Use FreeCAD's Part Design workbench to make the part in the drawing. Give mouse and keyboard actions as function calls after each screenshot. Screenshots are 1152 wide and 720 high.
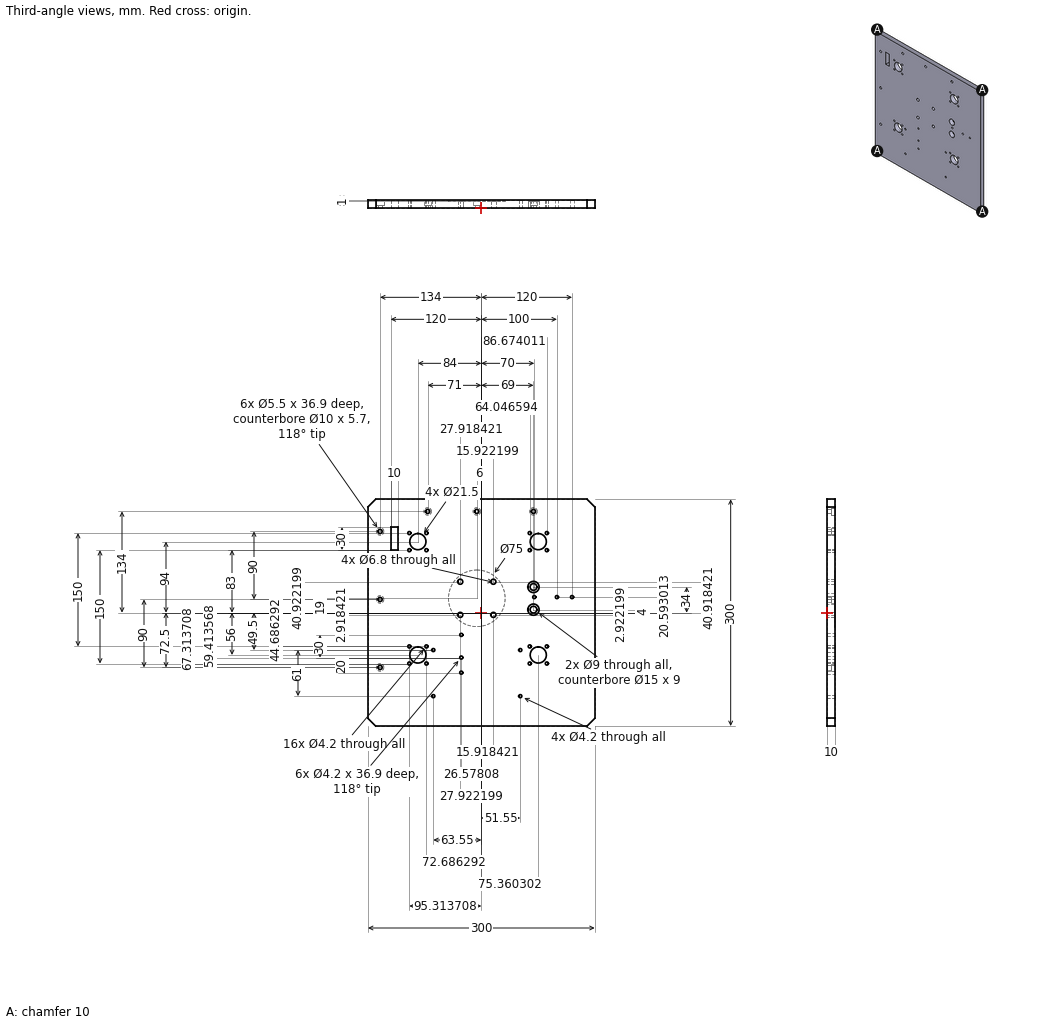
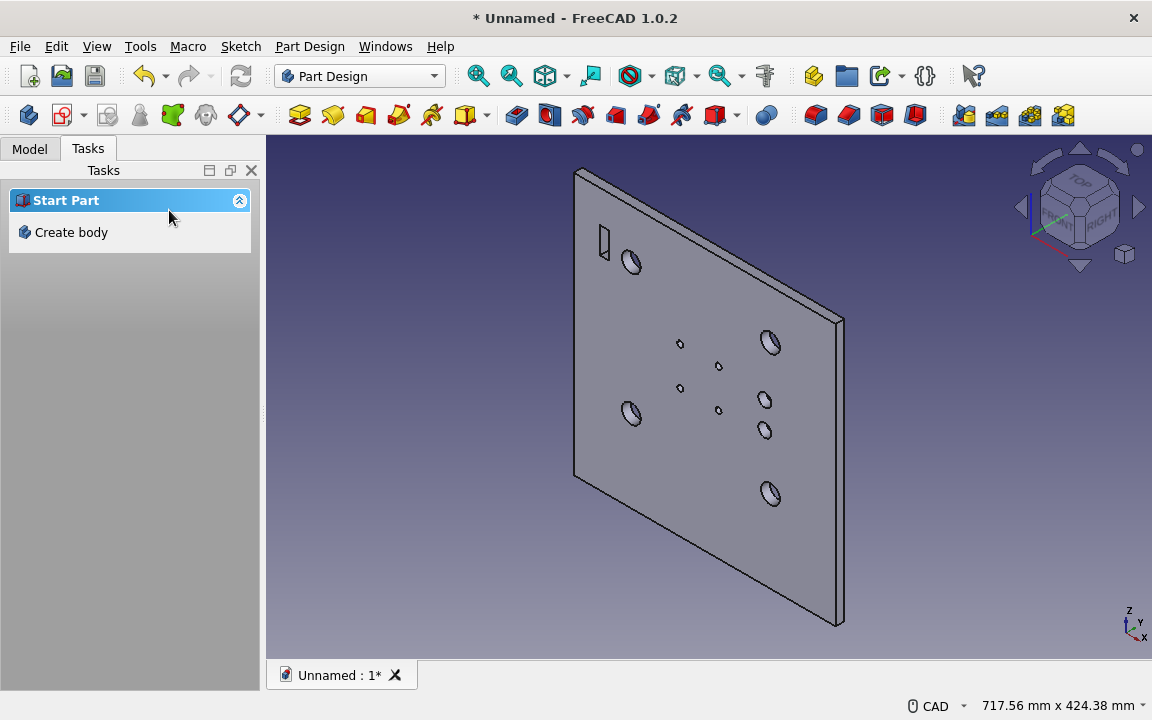
click(705, 485)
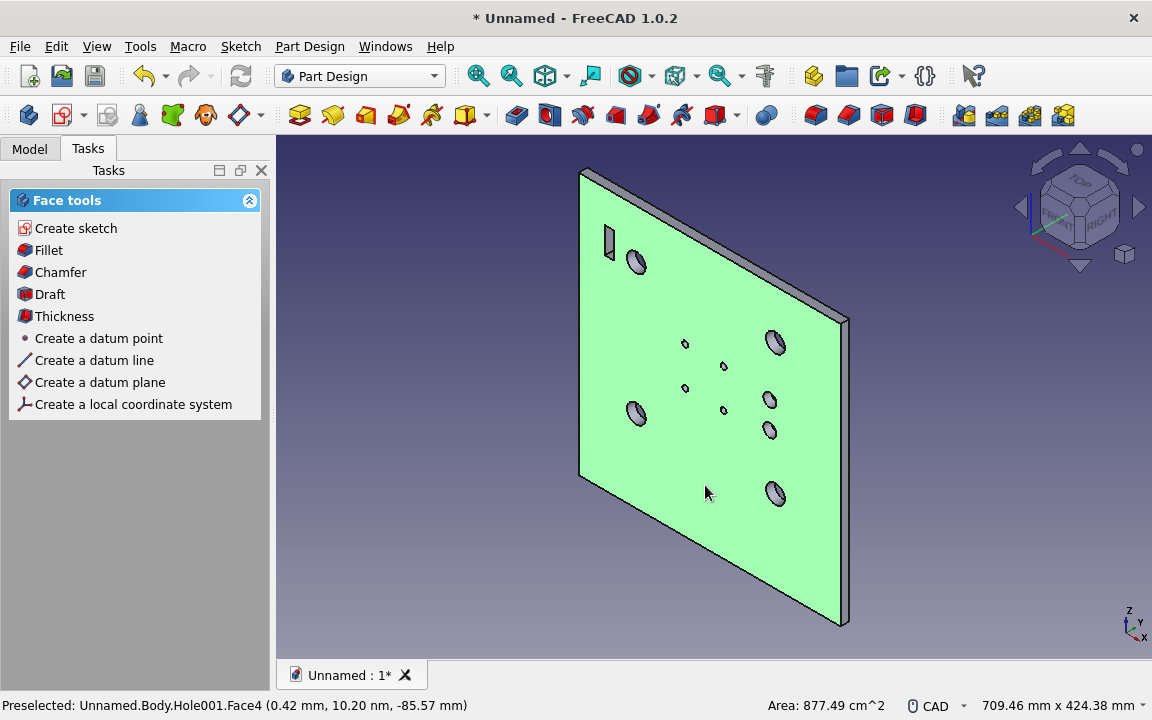
click(62, 116)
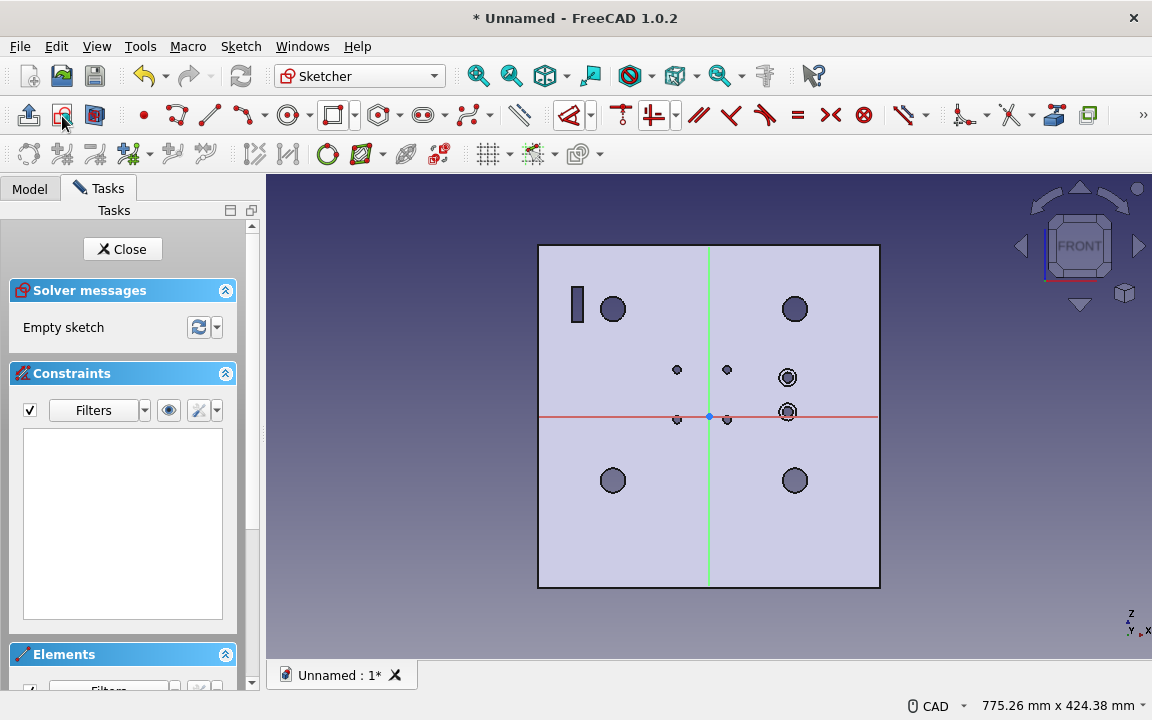
scroll(833, 351, up, 2)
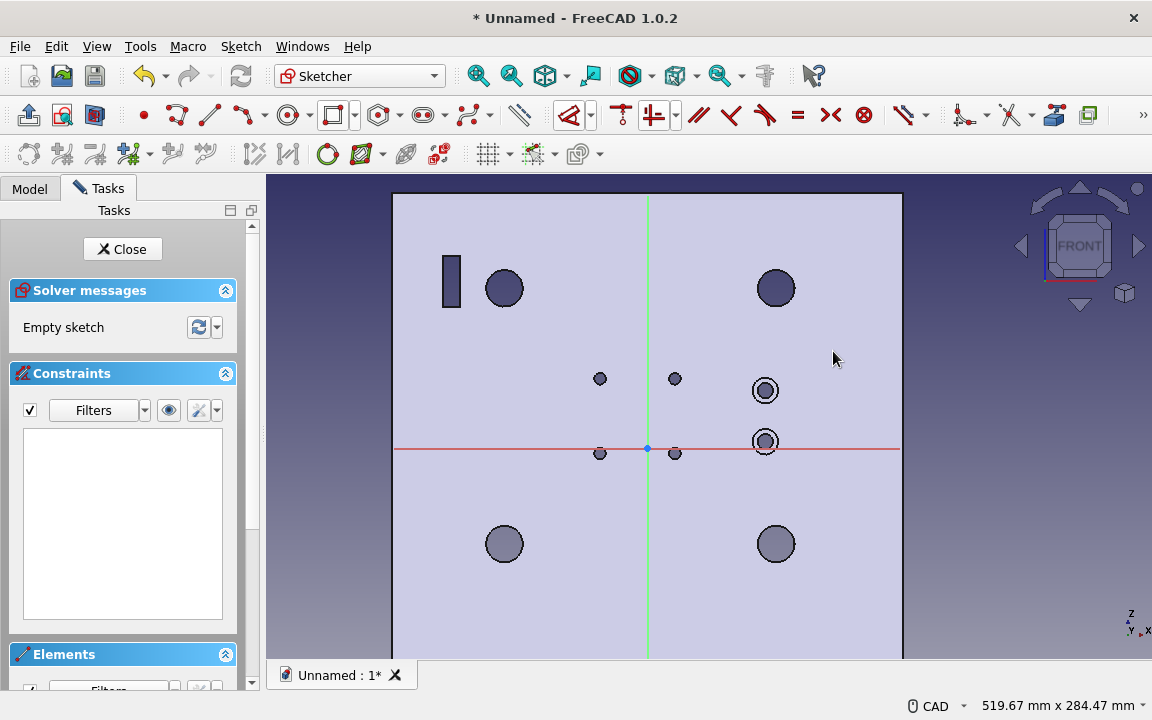
click(288, 116)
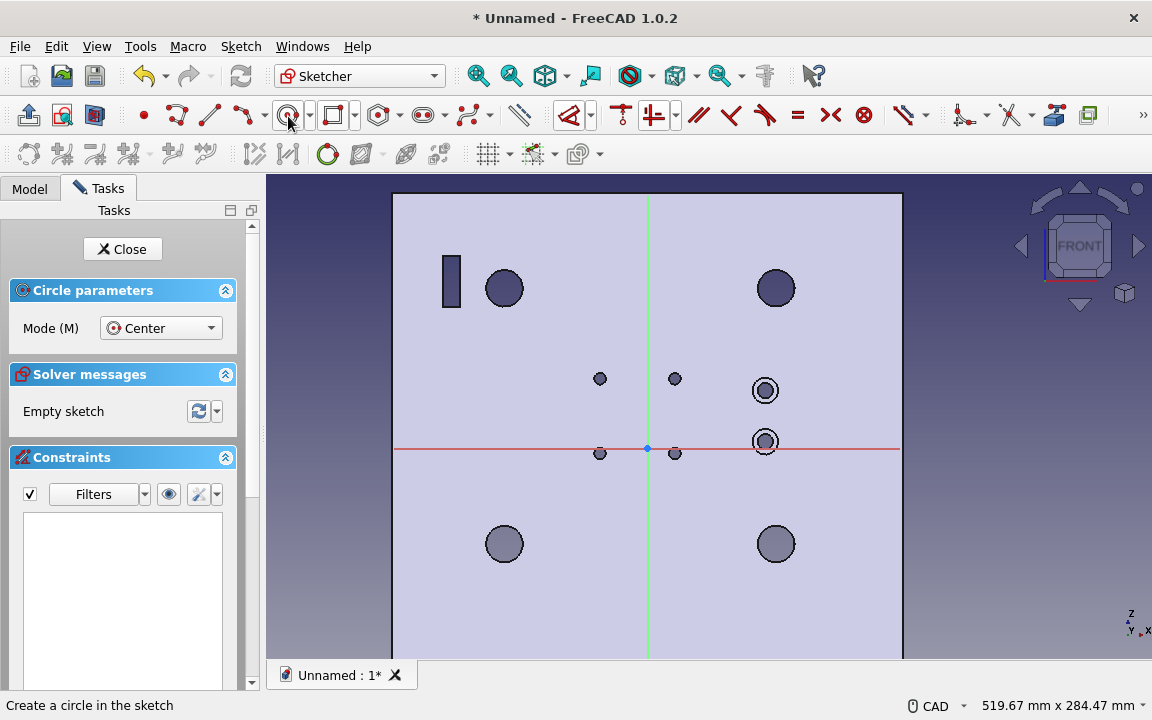
scroll(524, 525, up, 10)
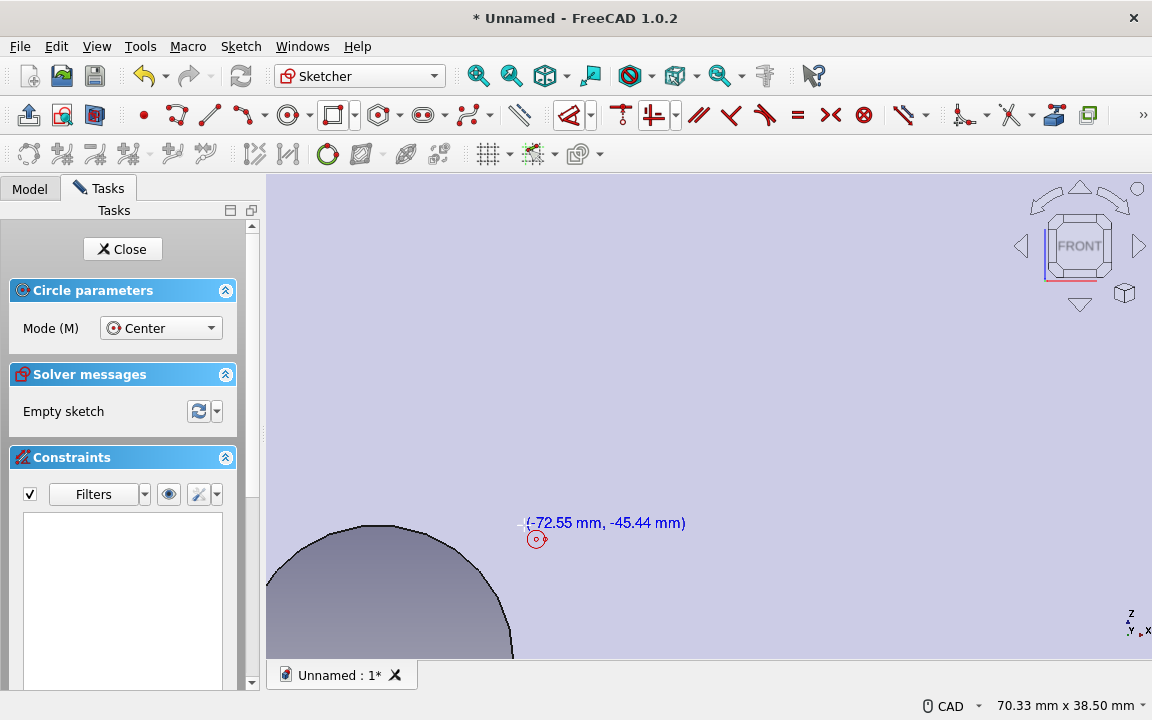
scroll(524, 526, down, 10)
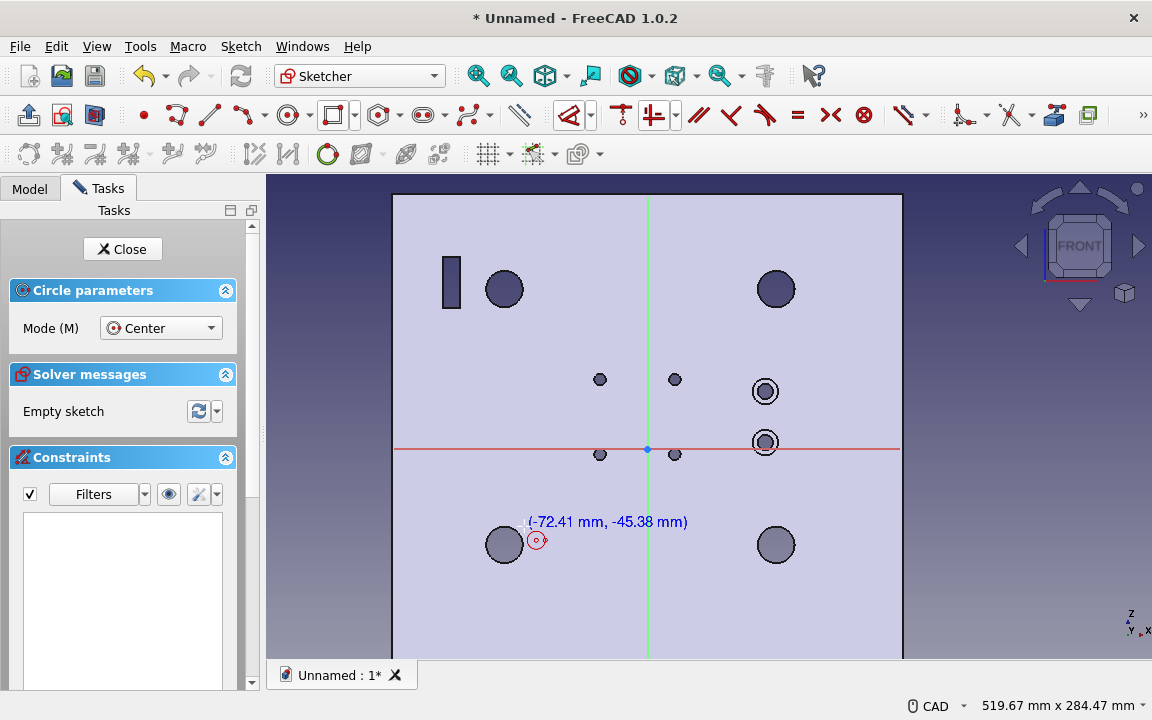
click(524, 526)
move(526, 523)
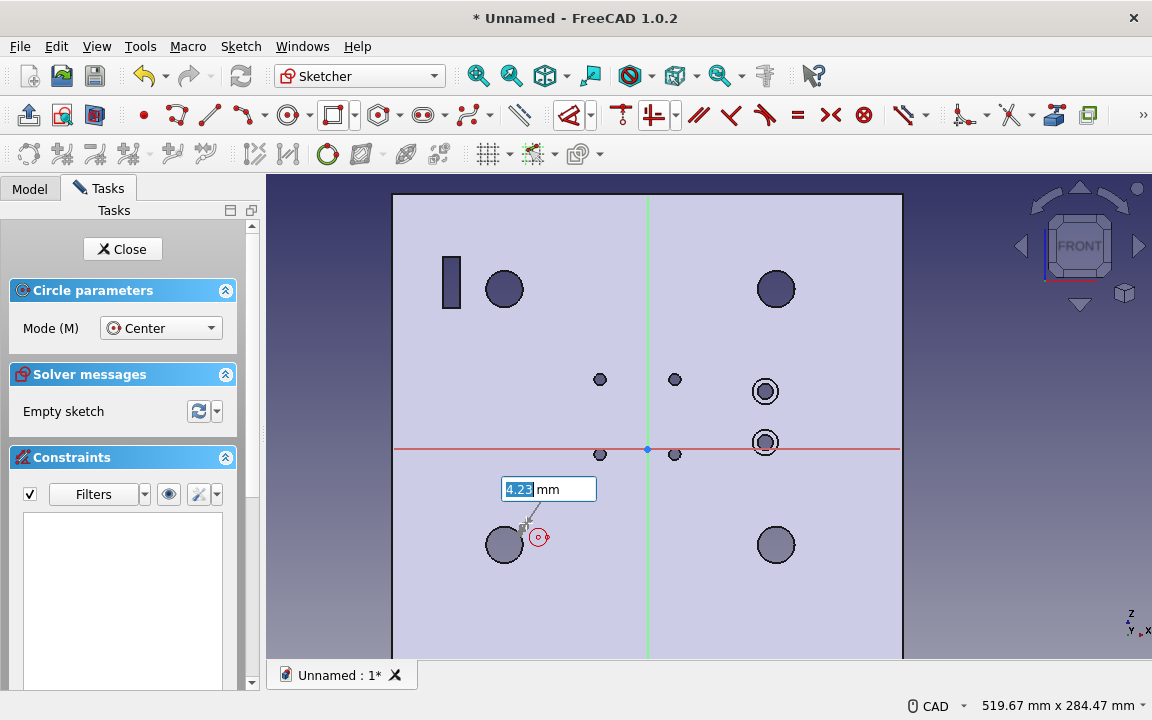
text(4.2)
key(Return)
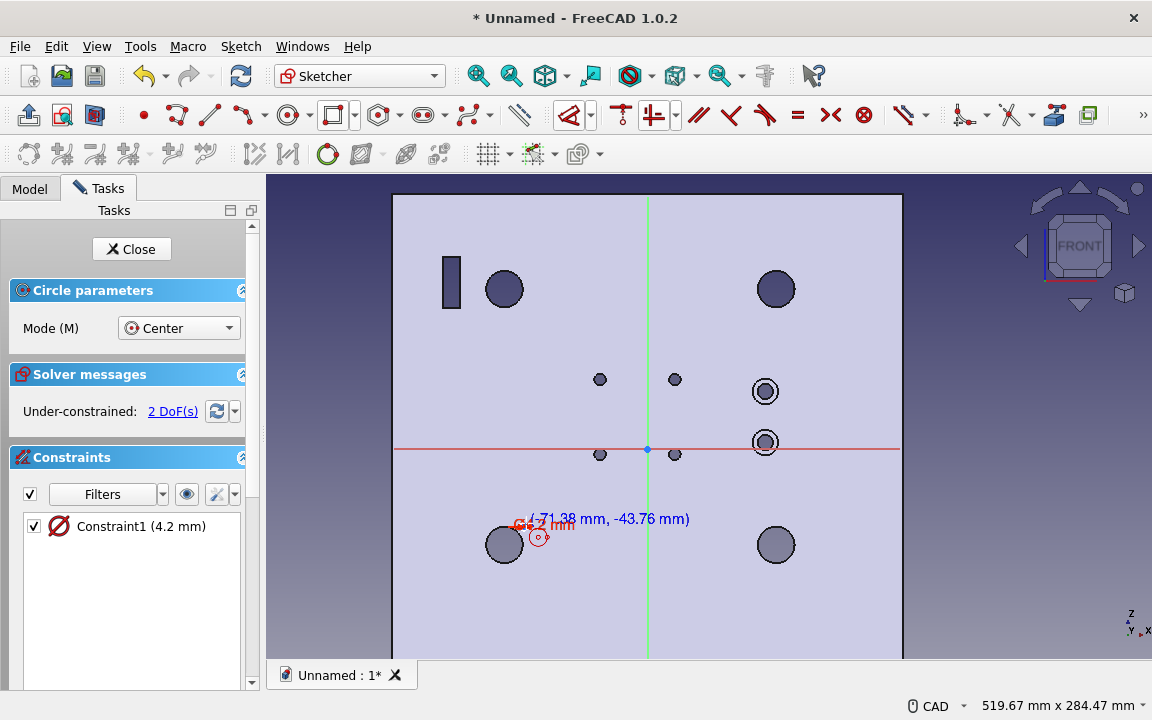
scroll(485, 526, up, 10)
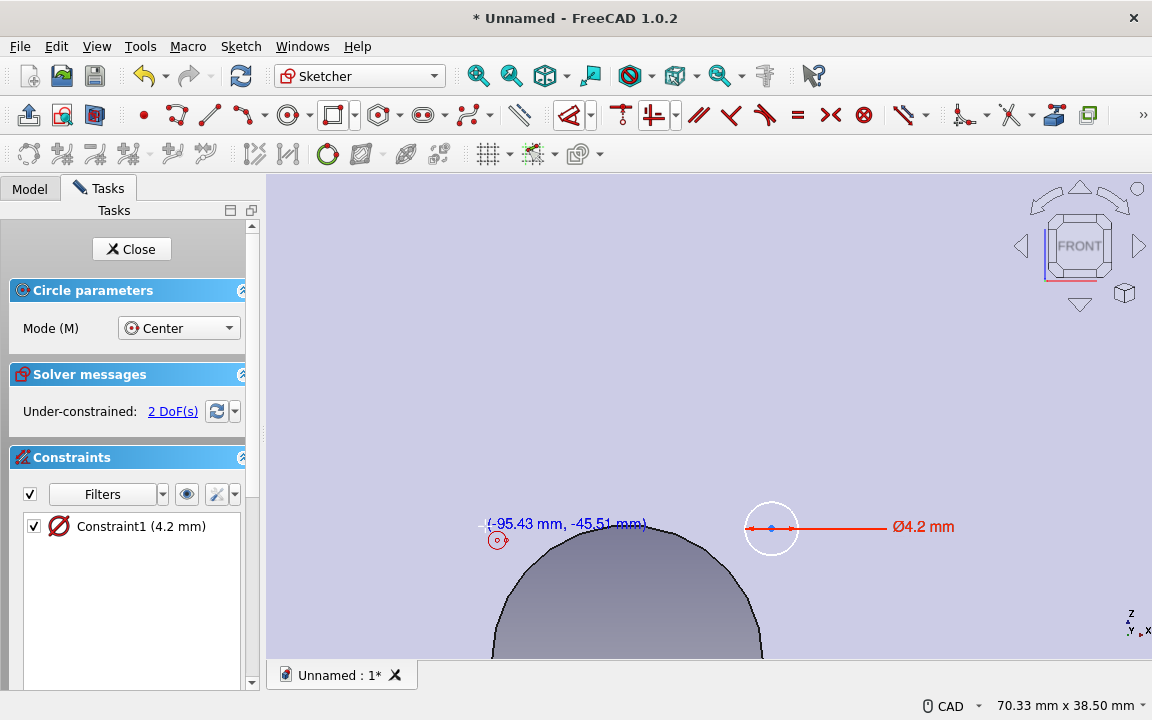
scroll(485, 526, down, 10)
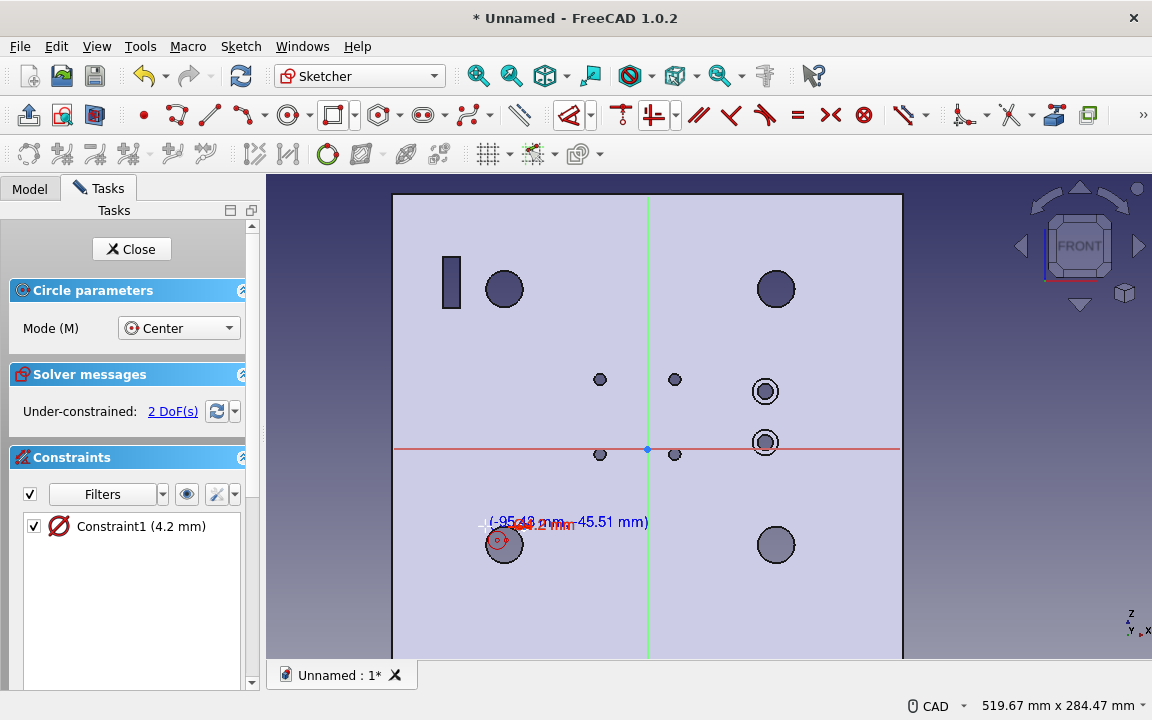
click(485, 526)
move(488, 523)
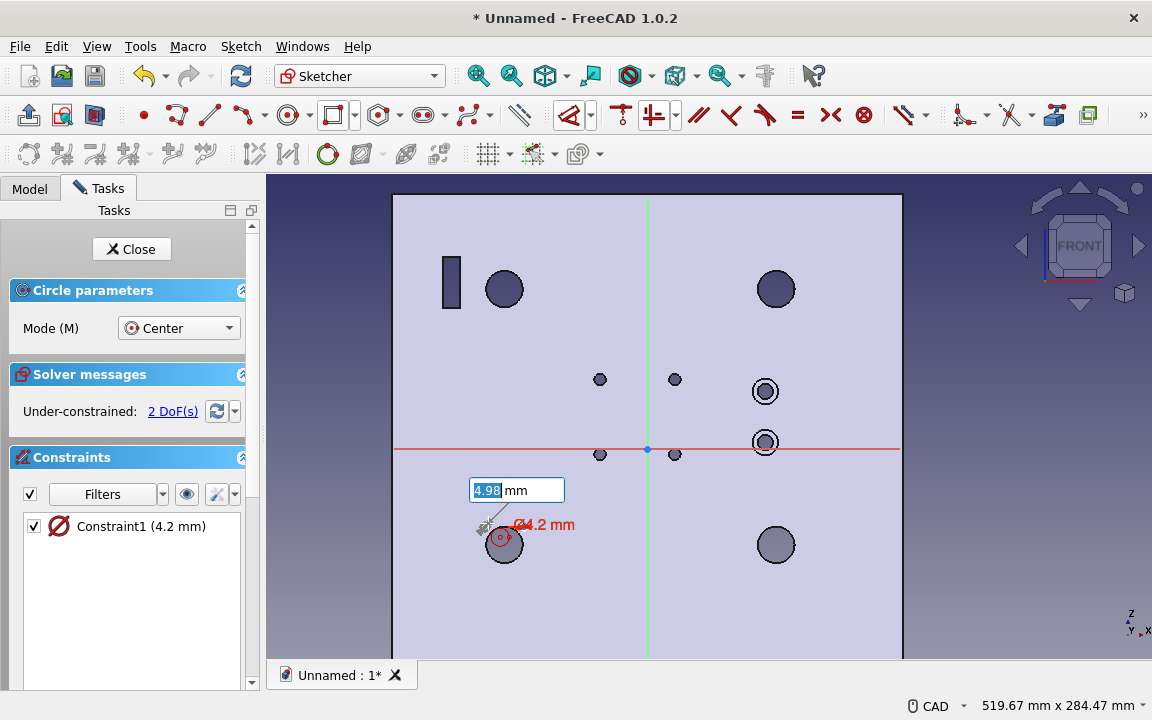
text(4.2)
key(Return)